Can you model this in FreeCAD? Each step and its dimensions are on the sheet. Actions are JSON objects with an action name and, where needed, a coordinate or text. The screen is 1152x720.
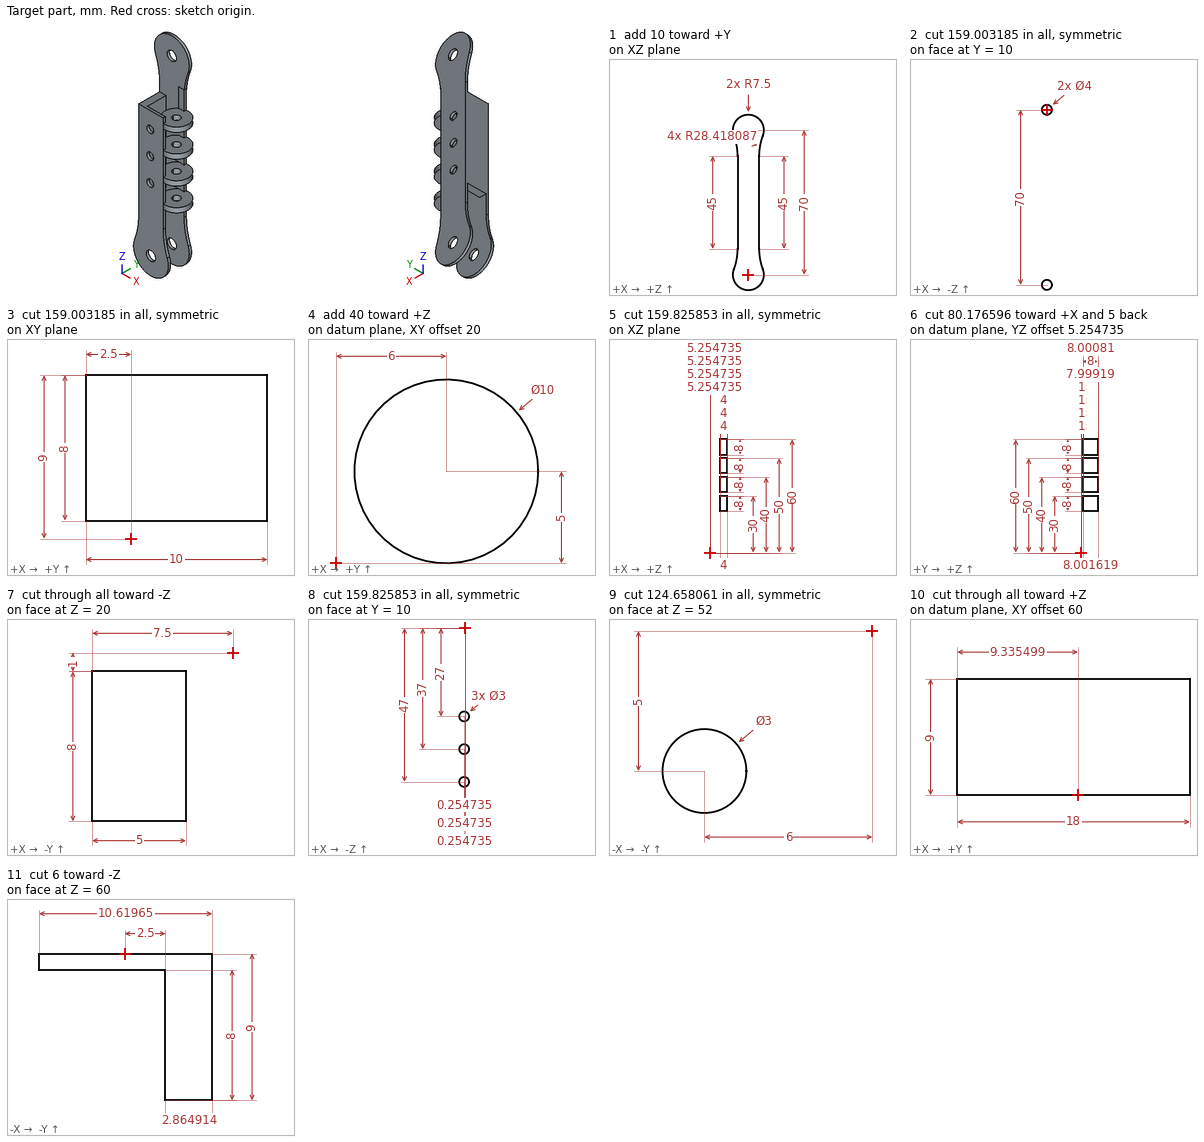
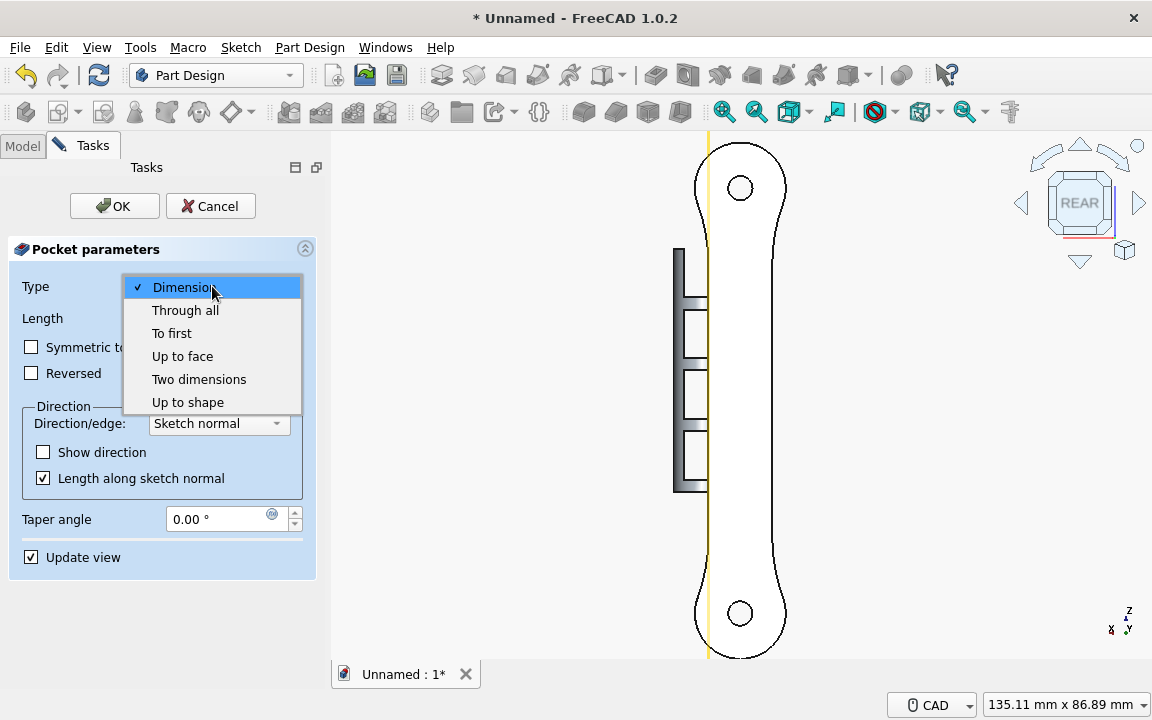
{"action": "left_click", "coordinate": [212, 380]}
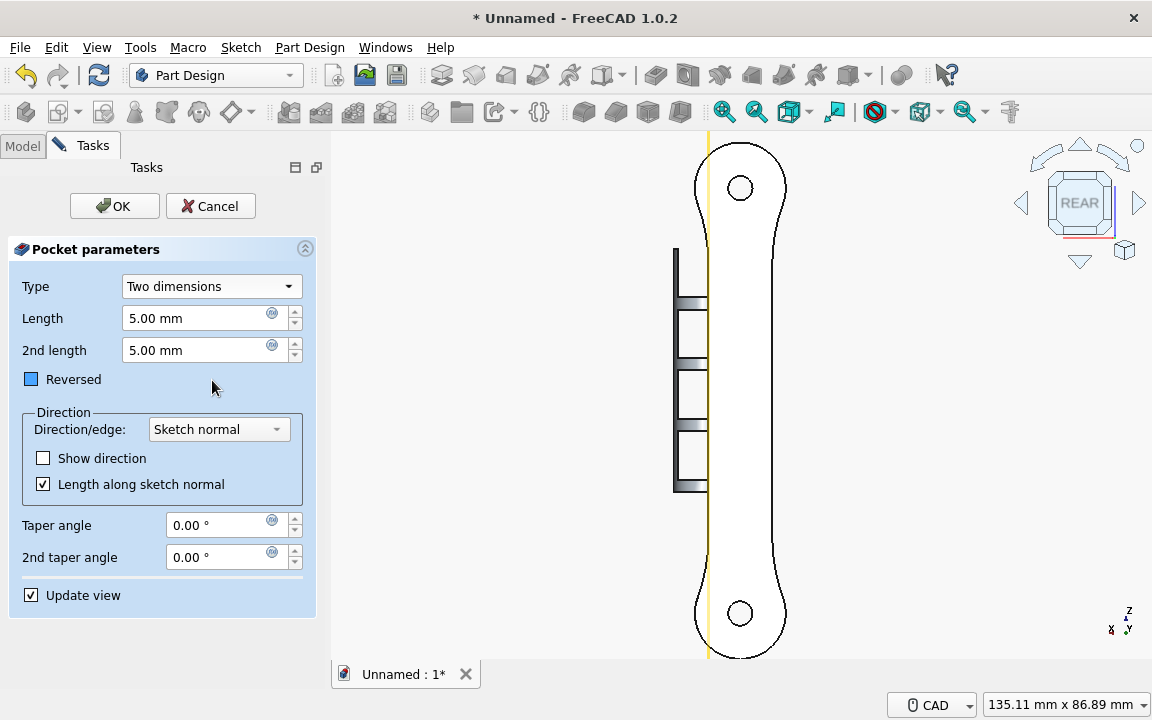
{"action": "triple_click", "coordinate": [204, 318]}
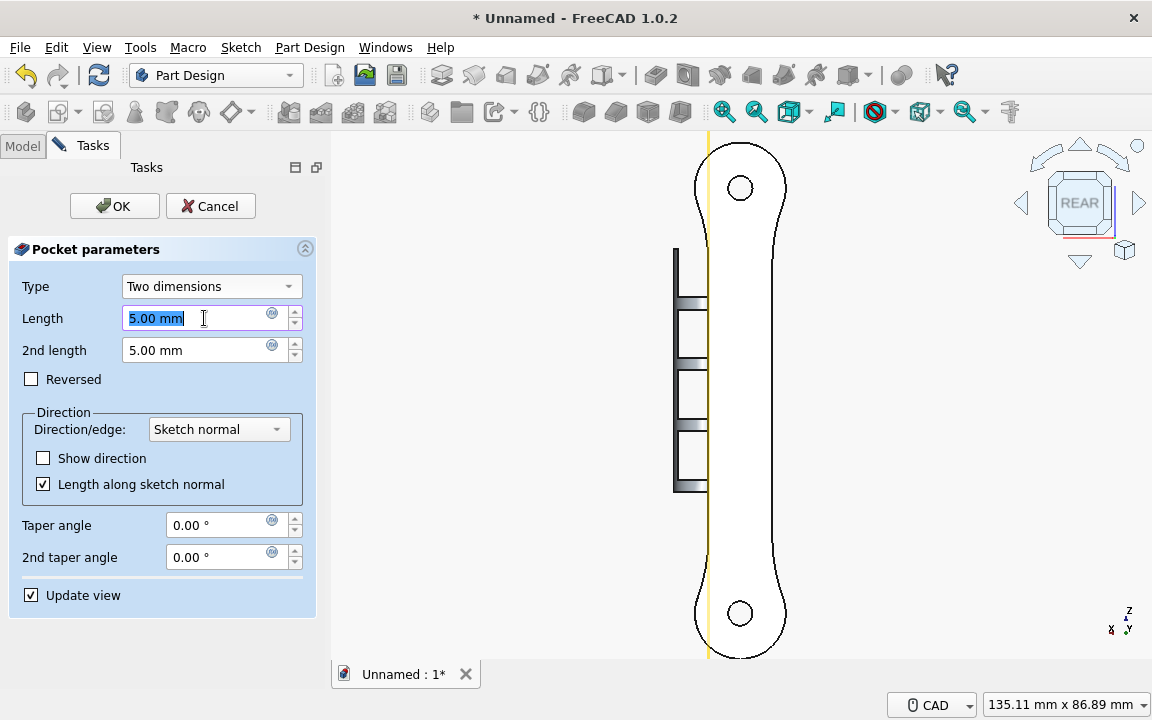
{"action": "type", "text": "80.176596"}
{"action": "key", "text": "Tab"}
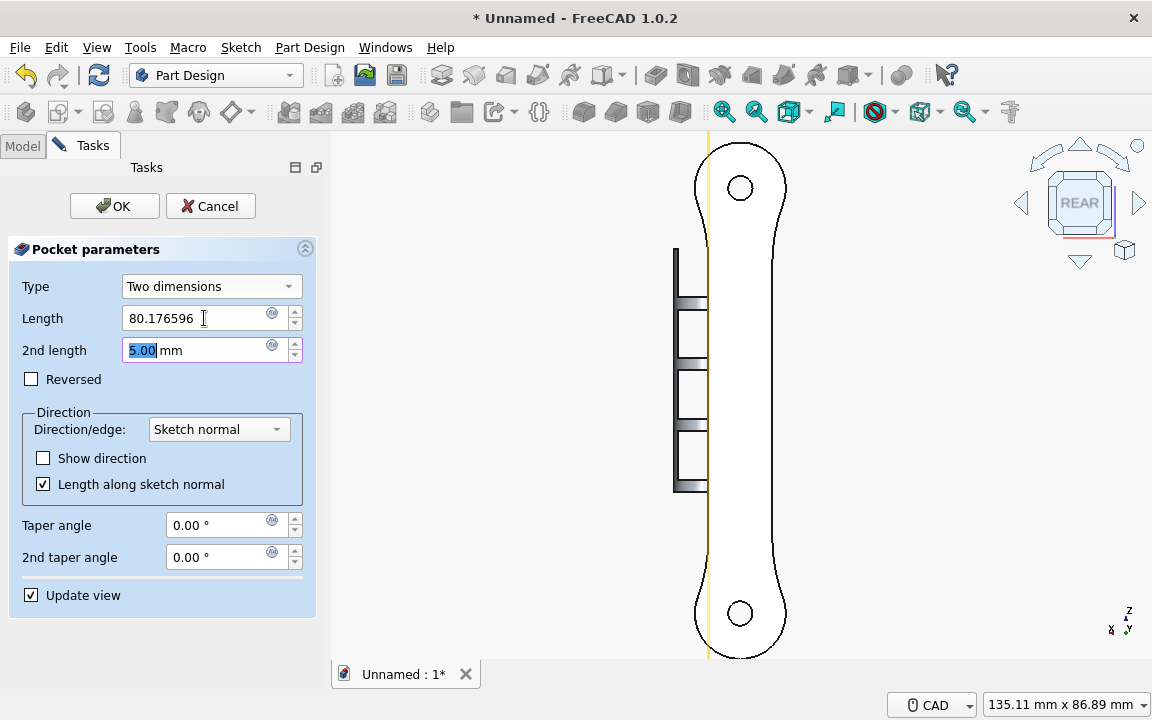
{"action": "type", "text": "5"}
{"action": "key", "text": "Tab"}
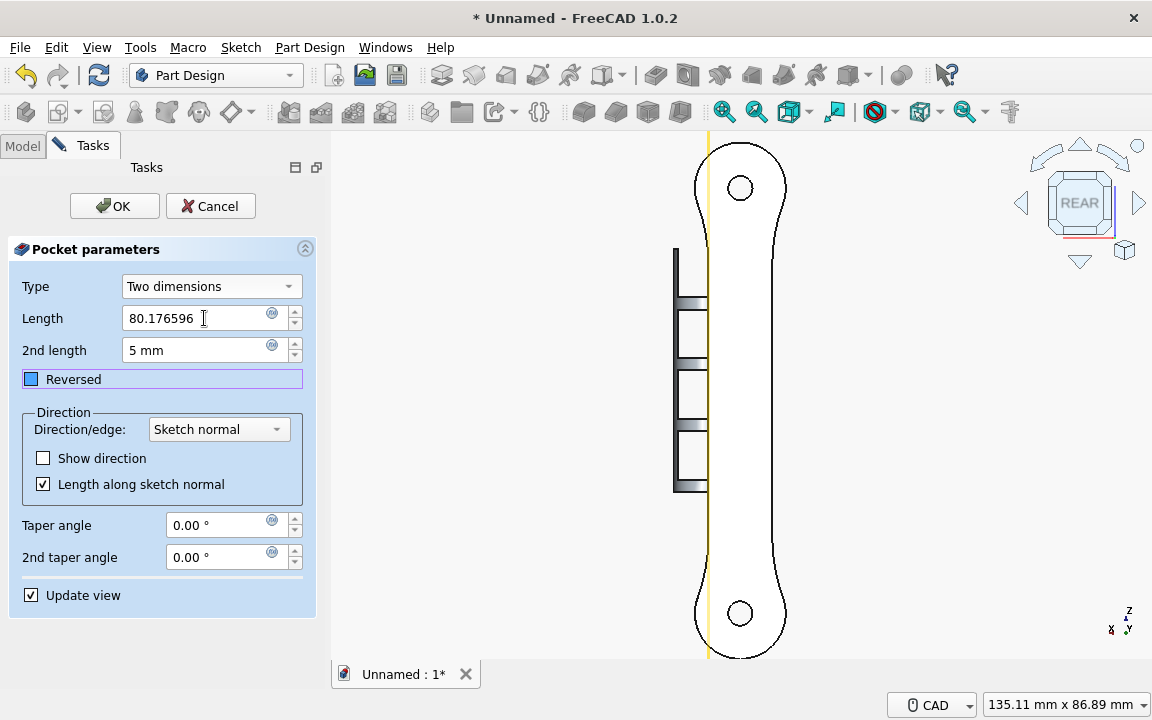
{"action": "left_click", "coordinate": [30, 379]}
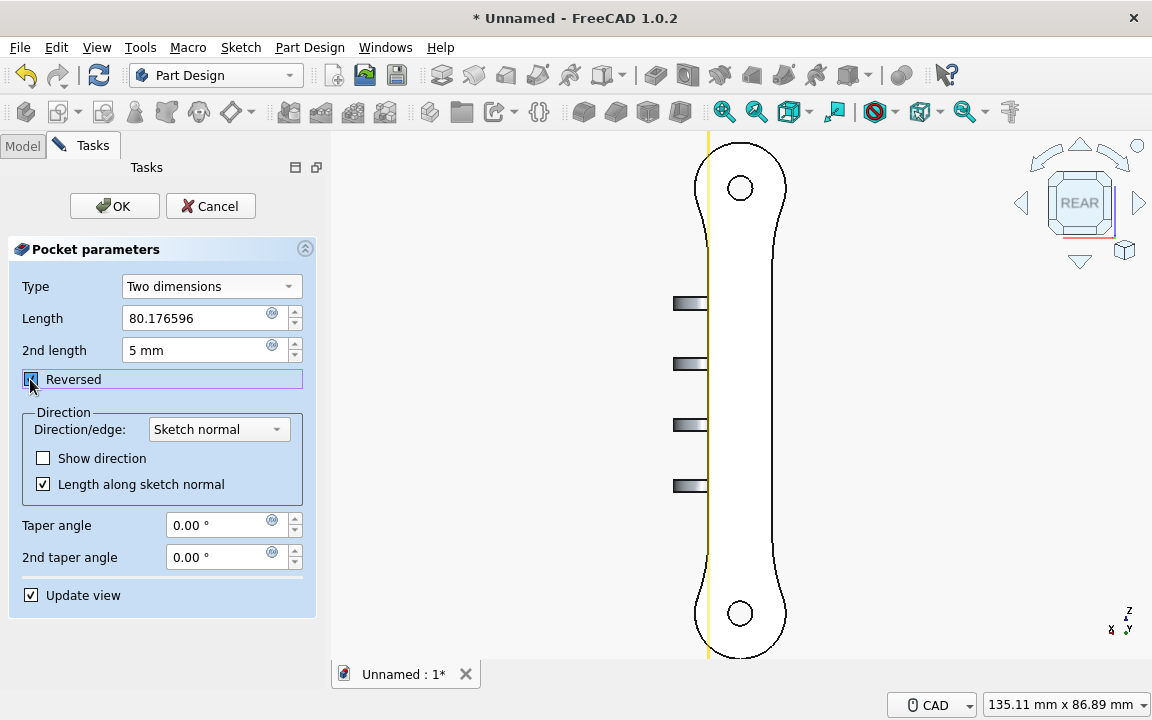
{"action": "left_click", "coordinate": [115, 206]}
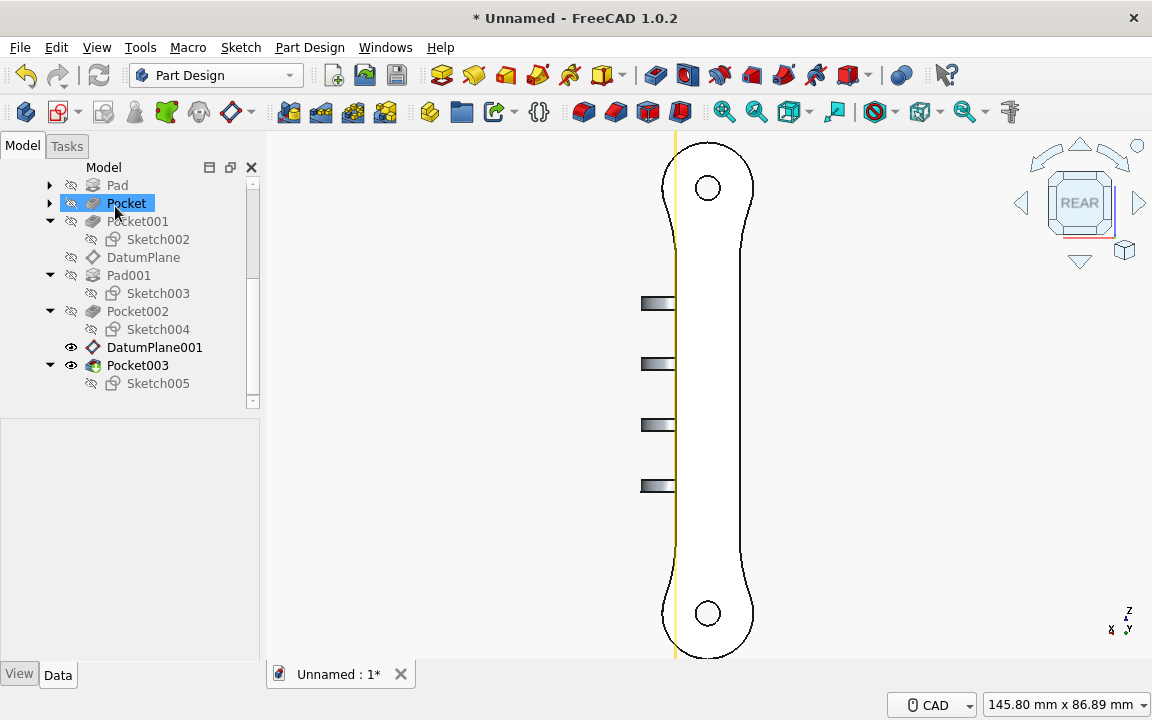
{"action": "left_click", "coordinate": [116, 347]}
{"action": "key", "text": "space"}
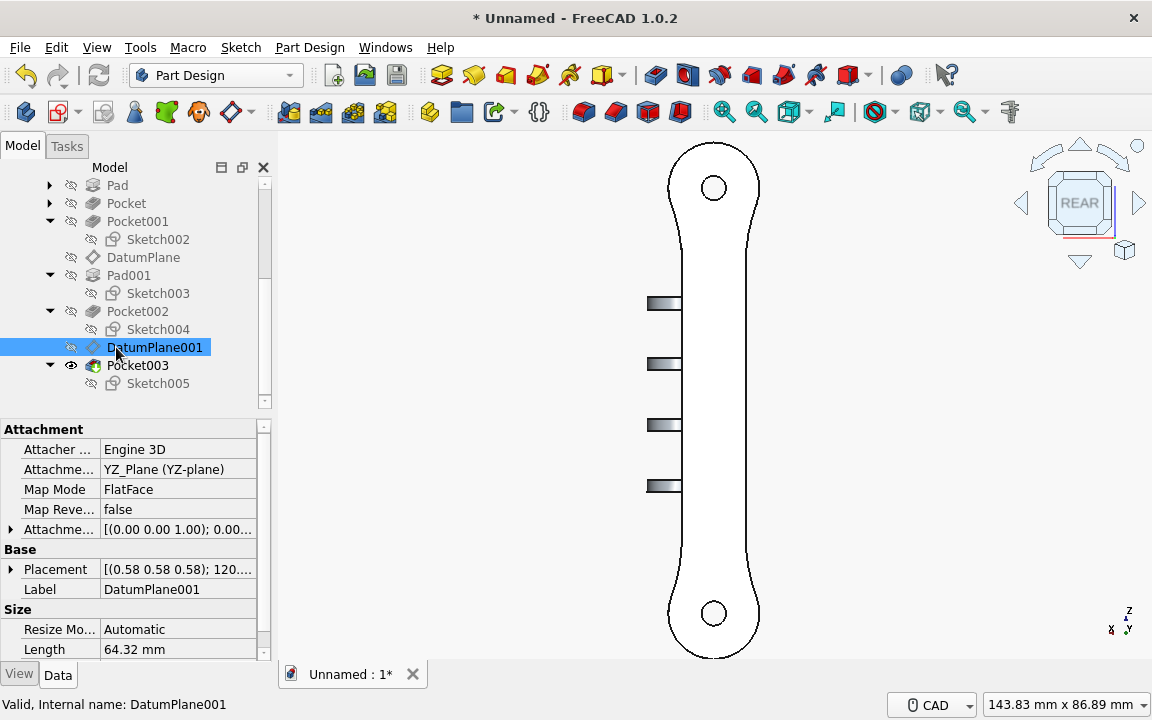
{"action": "key", "text": "5"}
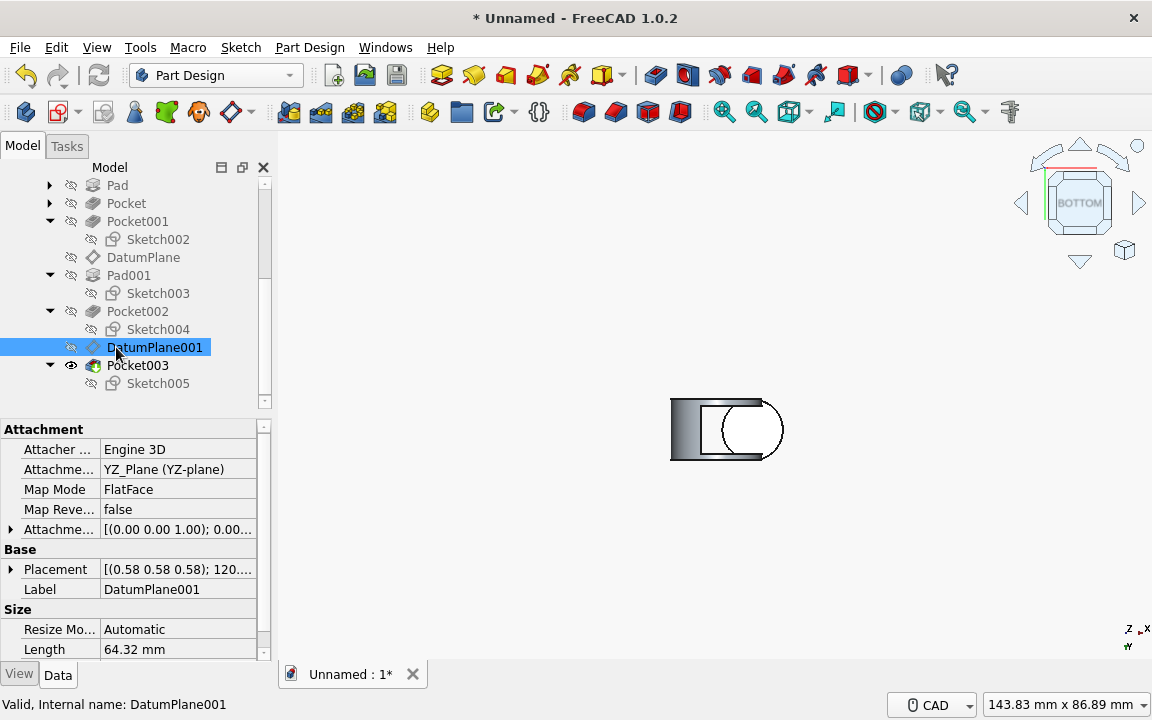
{"action": "left_click", "coordinate": [726, 112]}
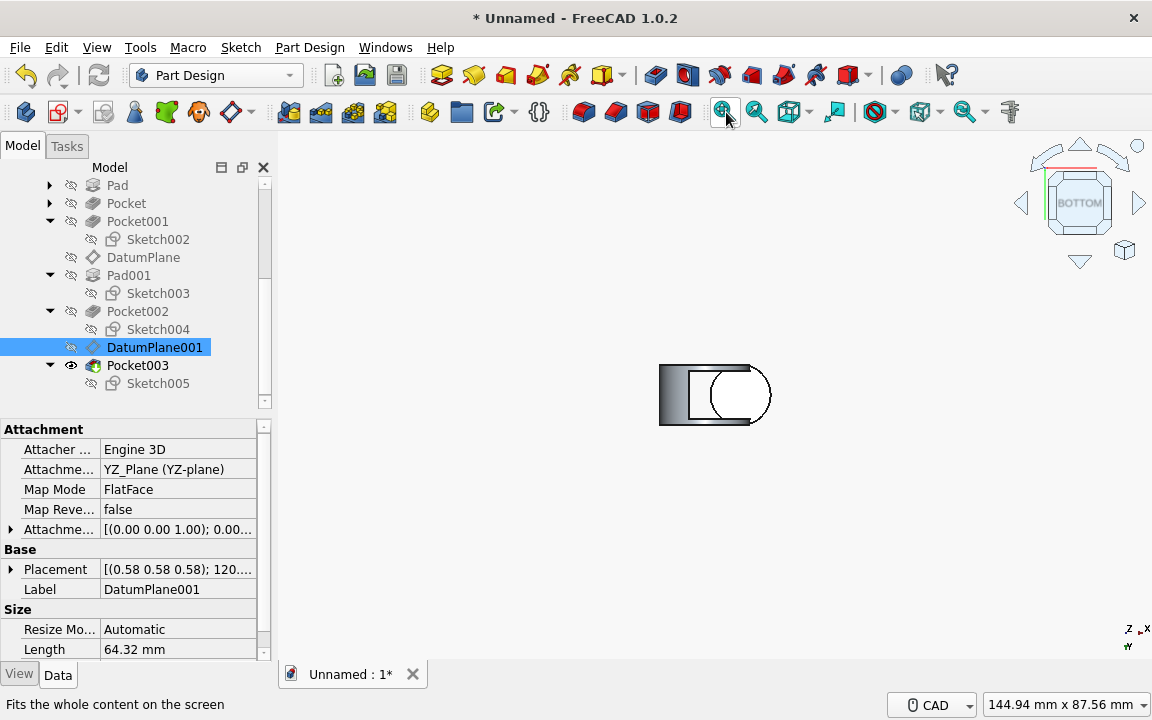
{"action": "left_click", "coordinate": [741, 394]}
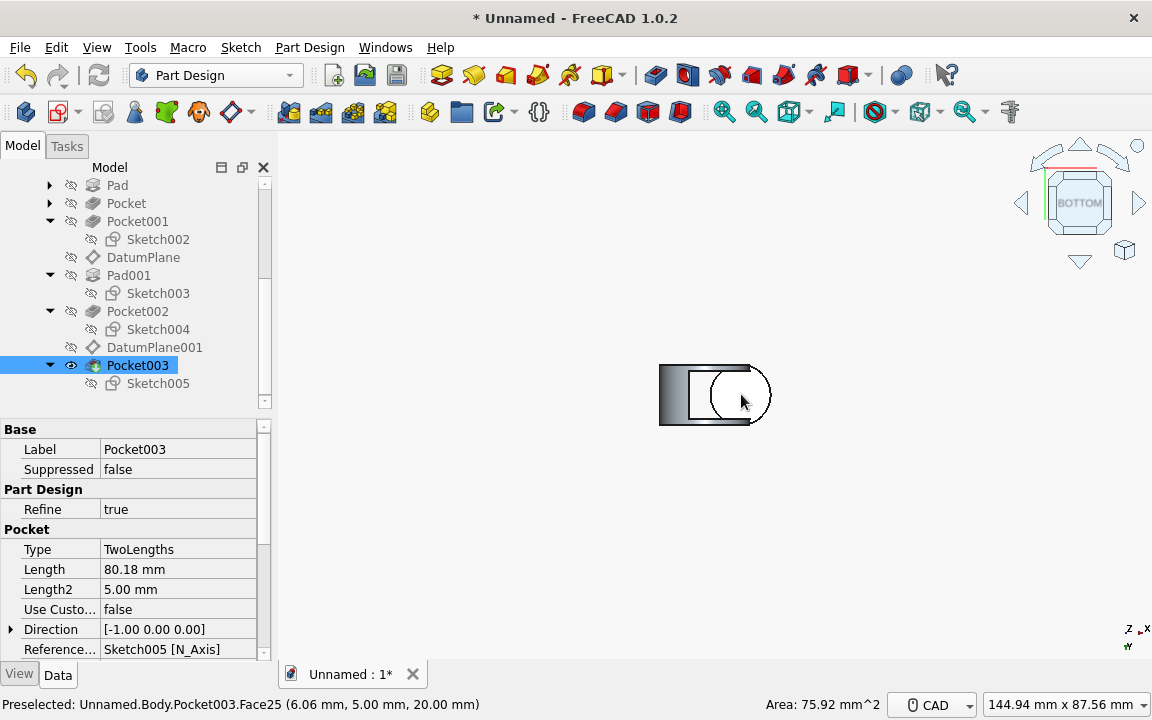
{"action": "left_click", "coordinate": [58, 112]}